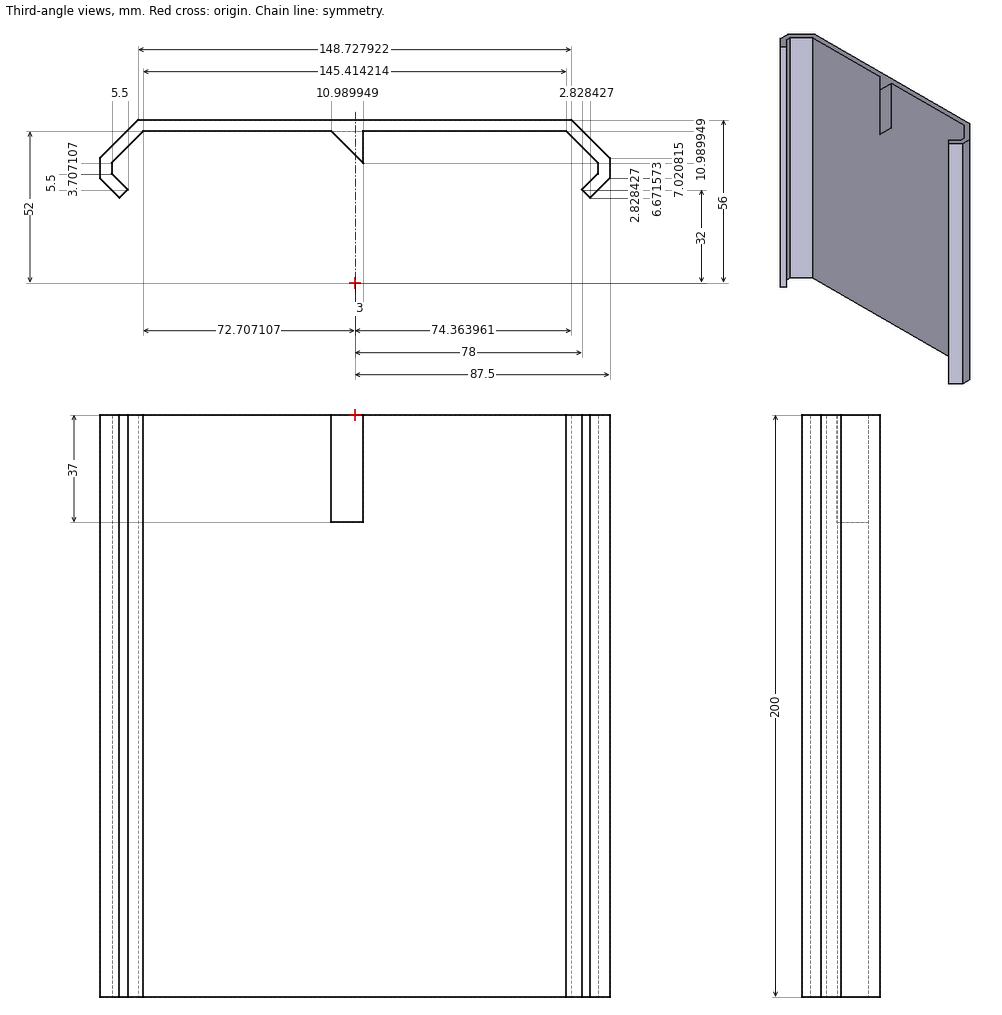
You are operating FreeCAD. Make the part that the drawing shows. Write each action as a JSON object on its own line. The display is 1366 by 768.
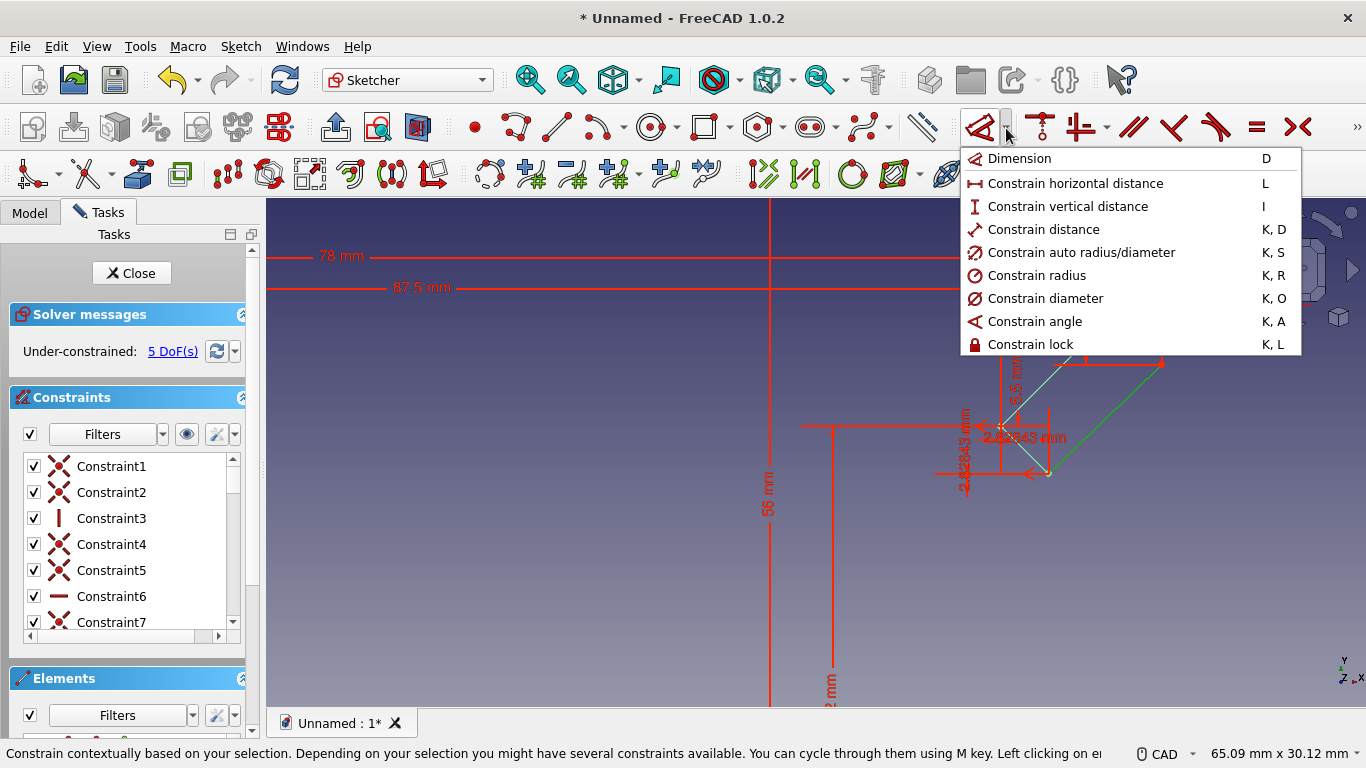
{"action": "left_click", "coordinate": [1131, 206]}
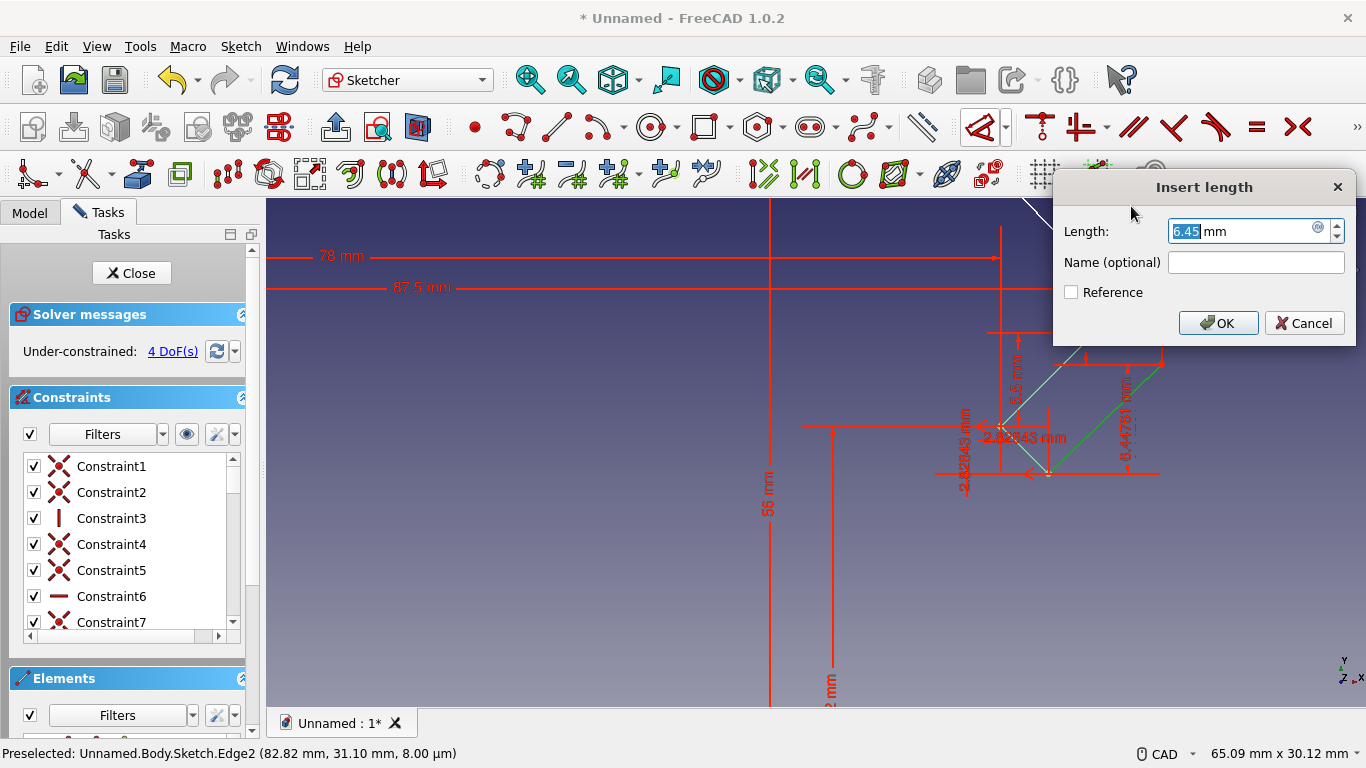
{"action": "type", "text": "6.671573"}
{"action": "key", "text": "Return"}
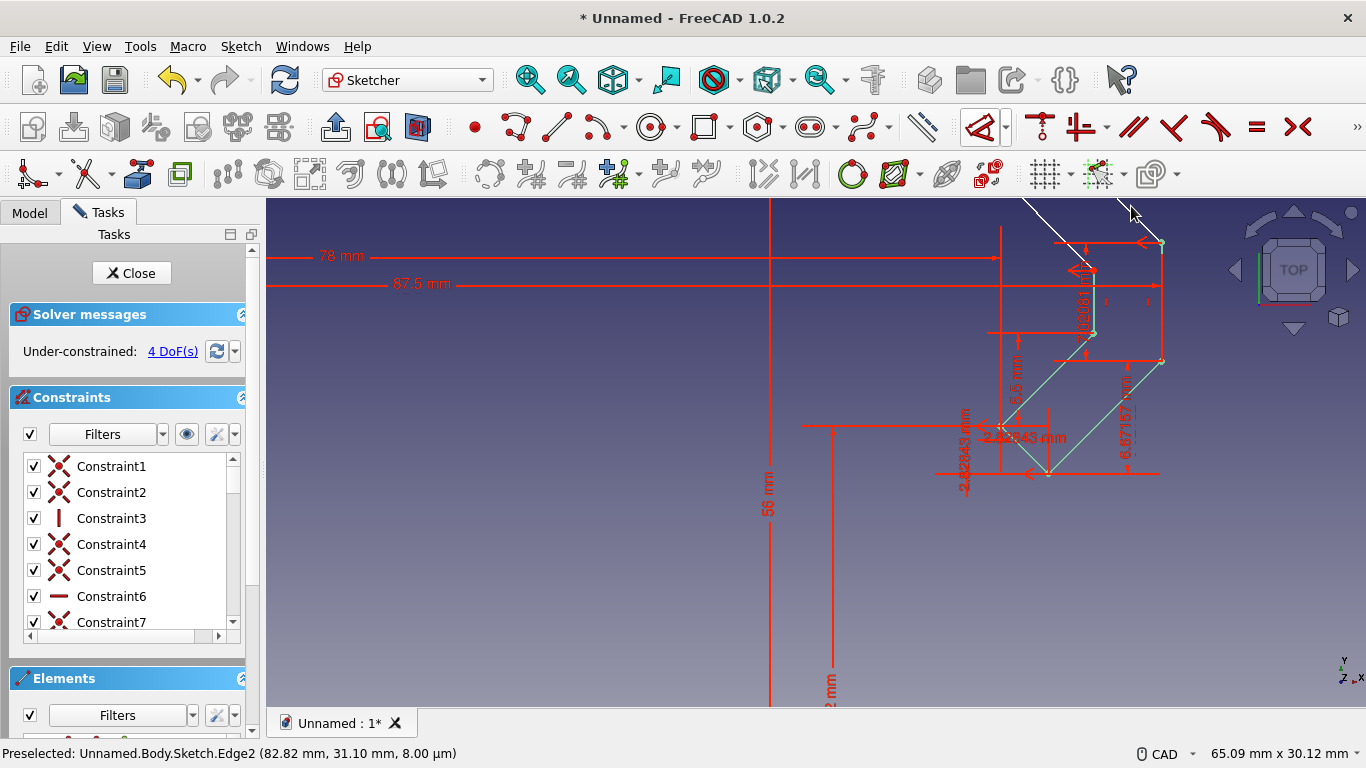
{"action": "scroll", "coordinate": [1017, 442], "scroll_direction": "down", "scroll_amount": 8}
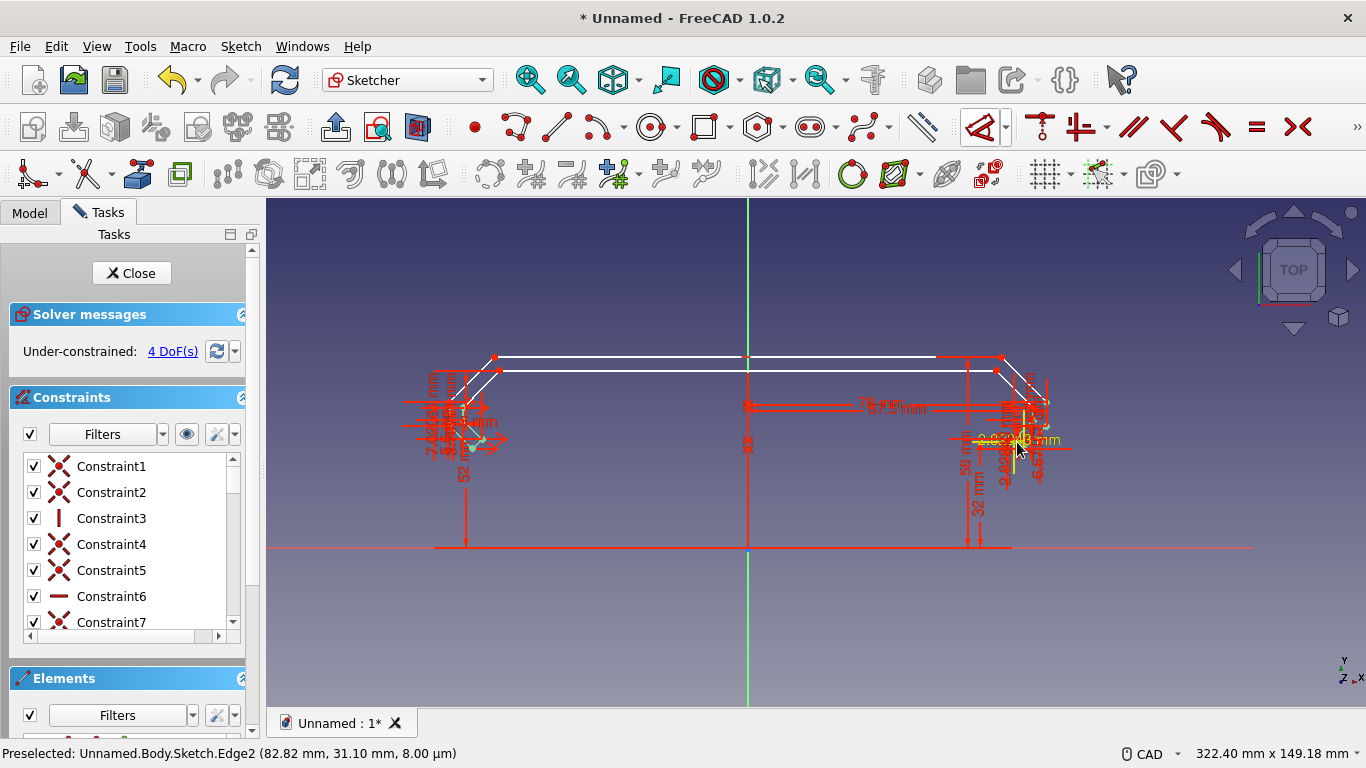
{"action": "left_click", "coordinate": [850, 357]}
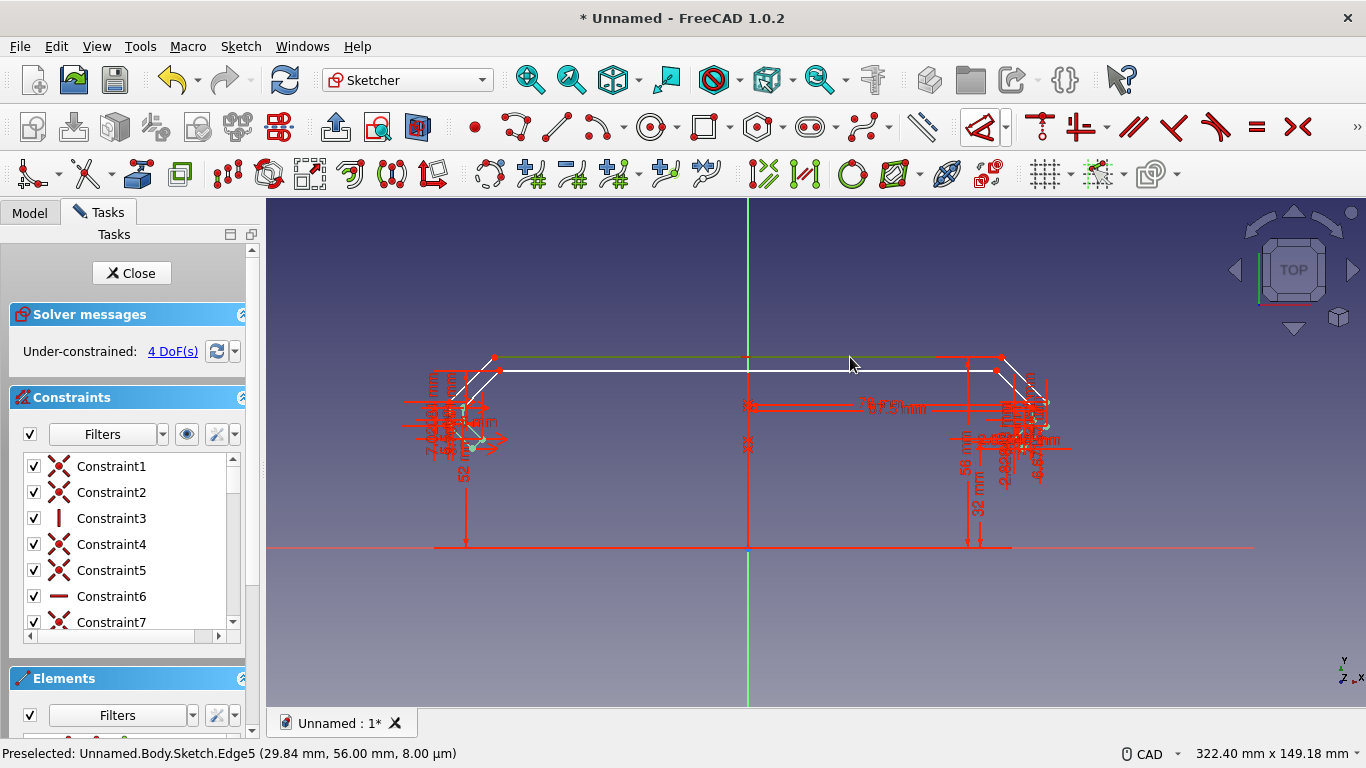
{"action": "key", "text": "l"}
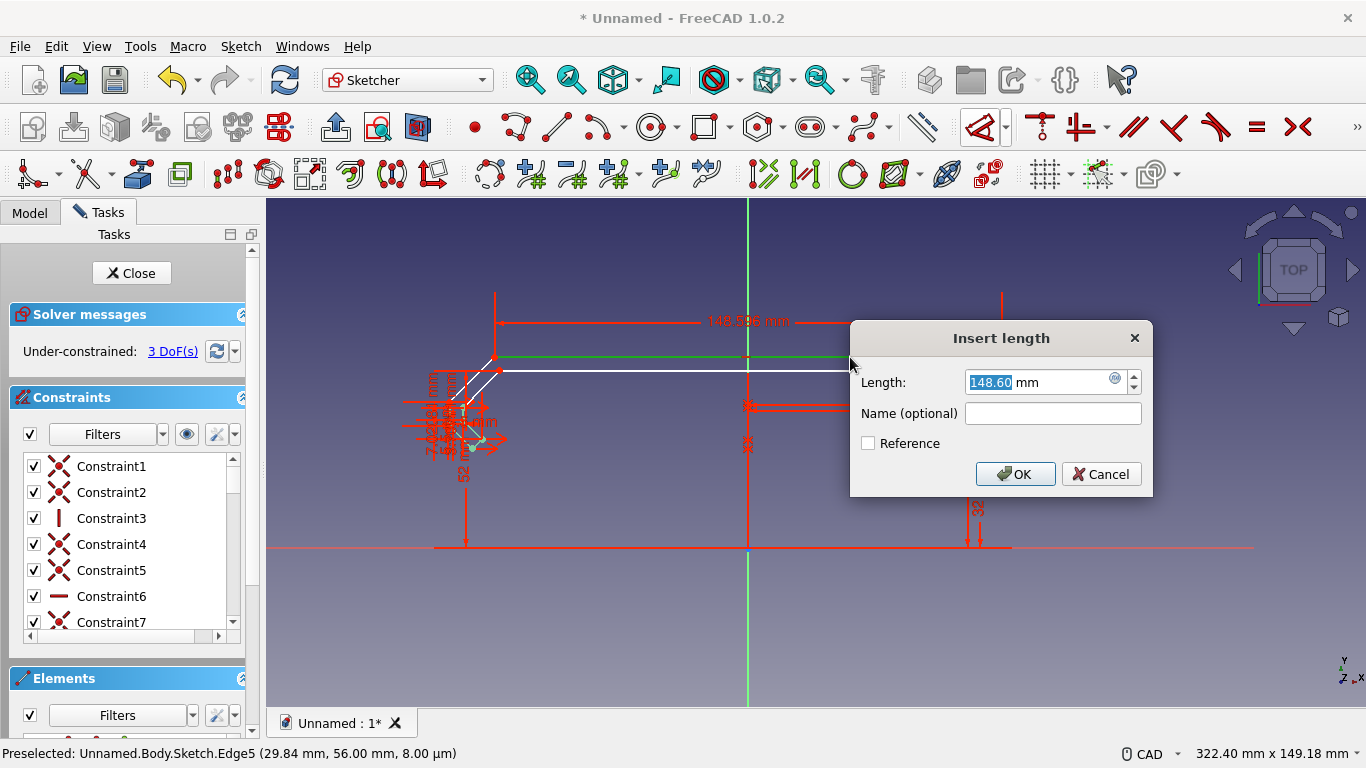
{"action": "type", "text": "148.727922"}
{"action": "key", "text": "Return"}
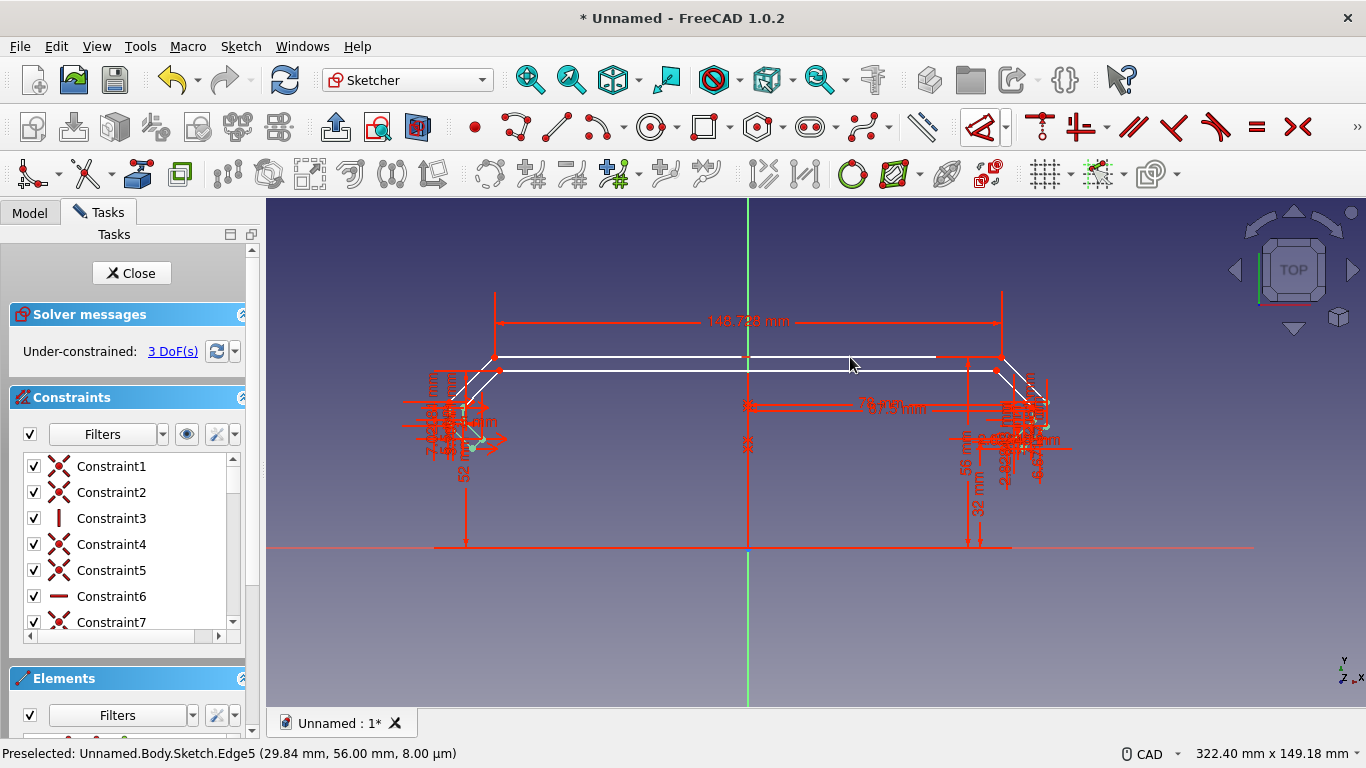
{"action": "left_click", "coordinate": [649, 371]}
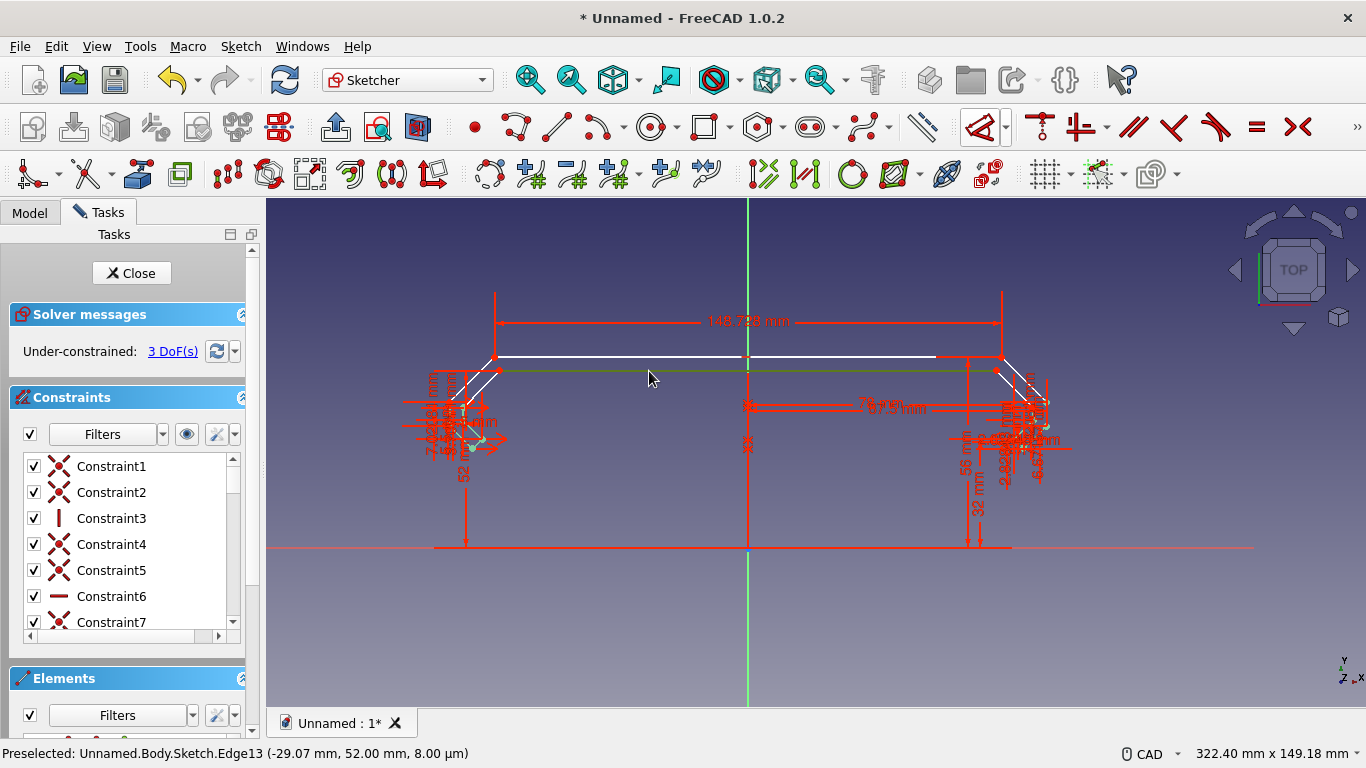
{"action": "key", "text": "l"}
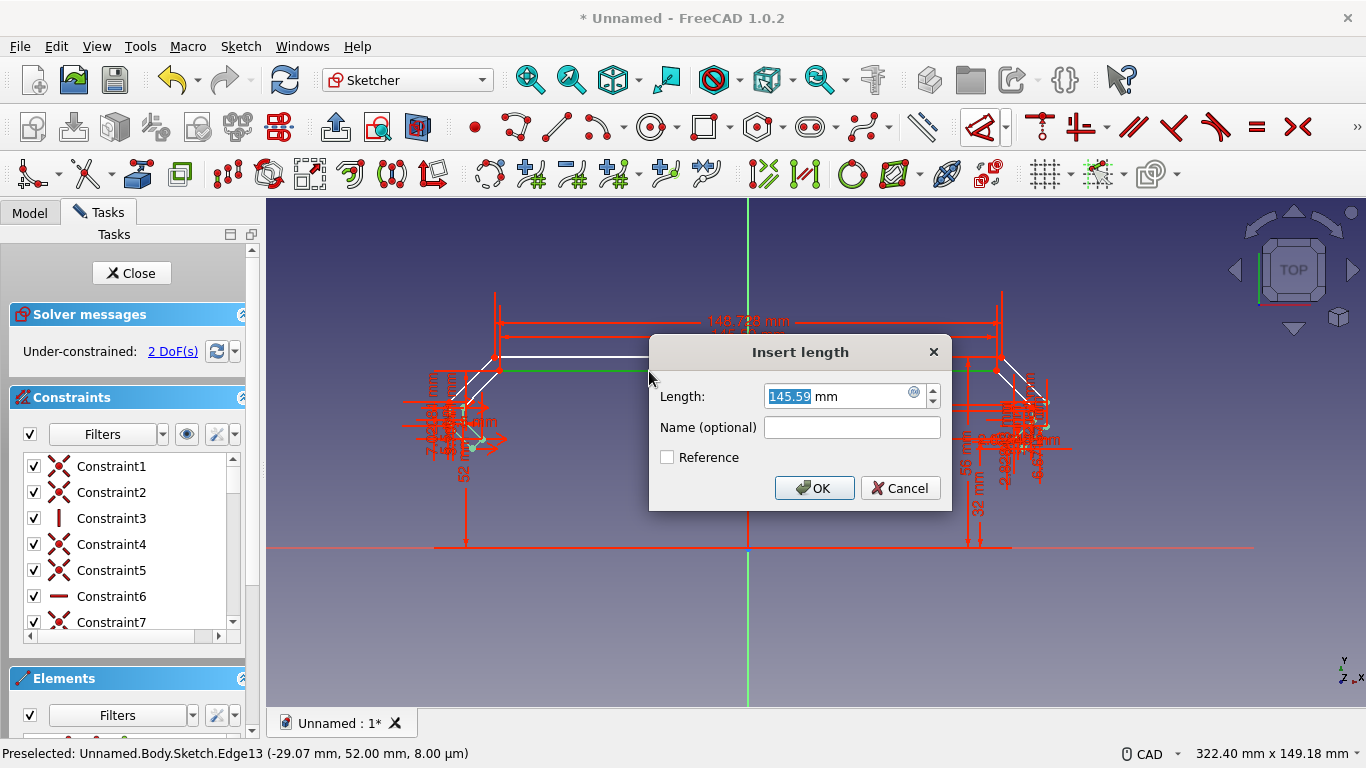
{"action": "type", "text": "145.414214"}
{"action": "key", "text": "Return"}